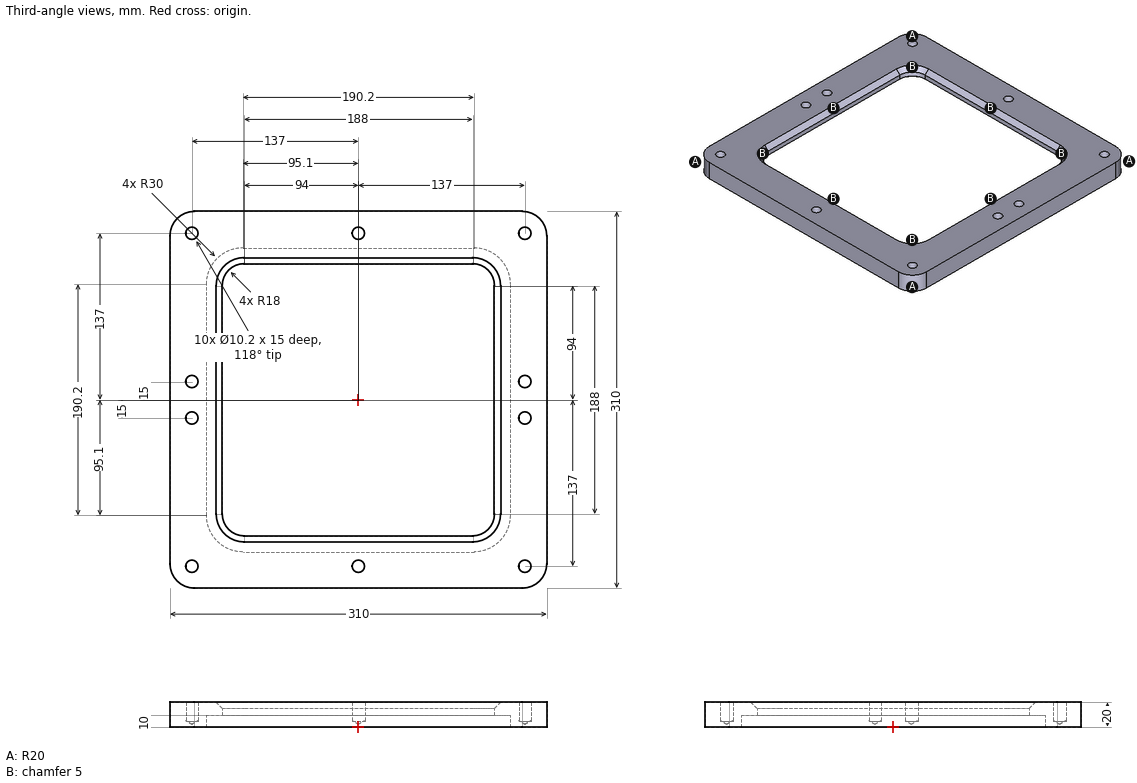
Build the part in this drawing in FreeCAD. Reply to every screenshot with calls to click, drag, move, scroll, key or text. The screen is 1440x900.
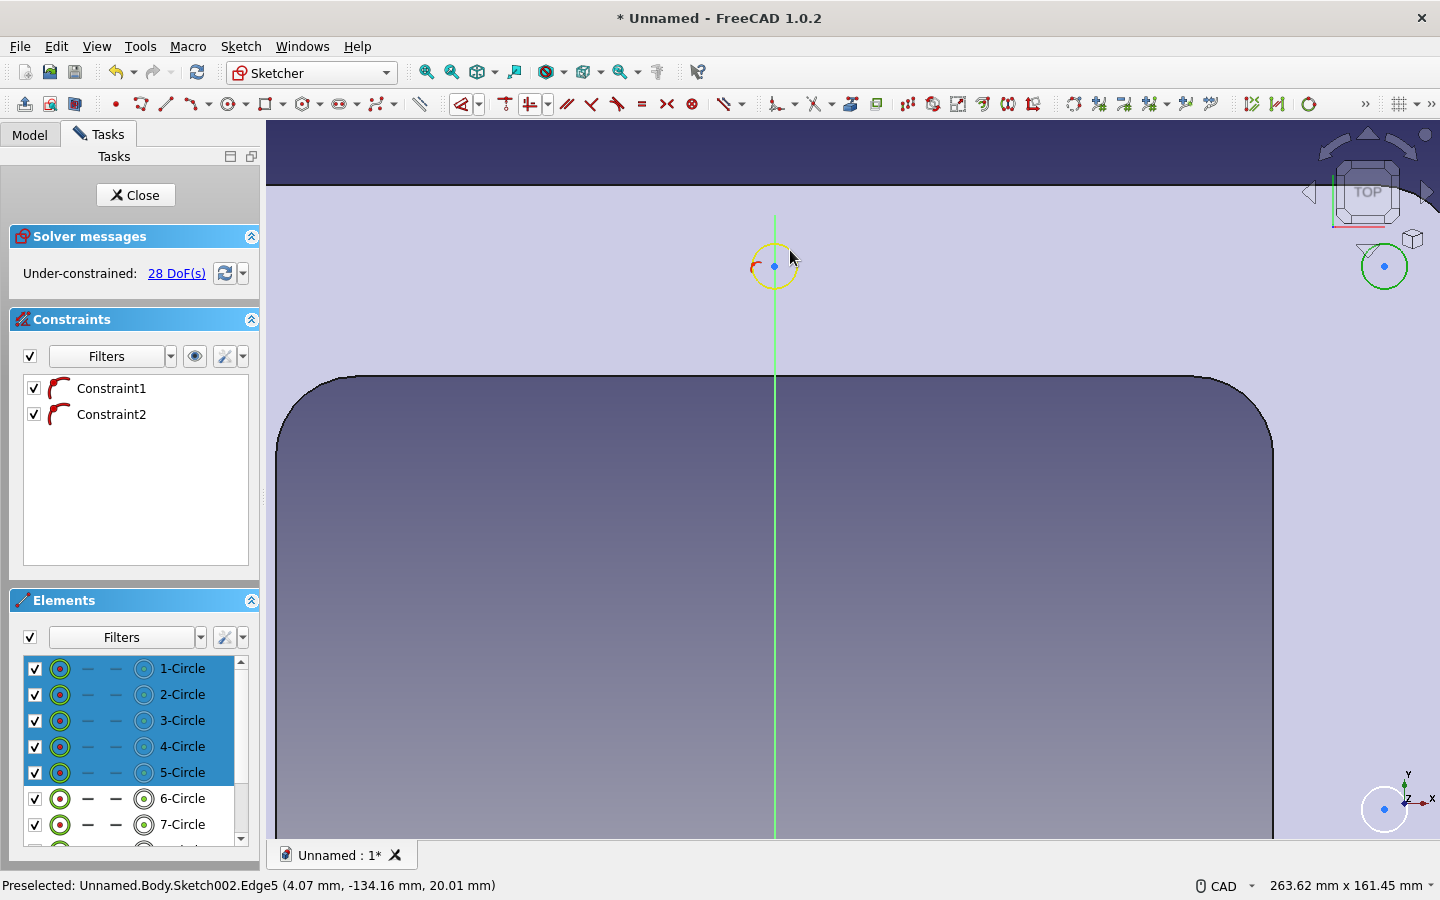
click(790, 250)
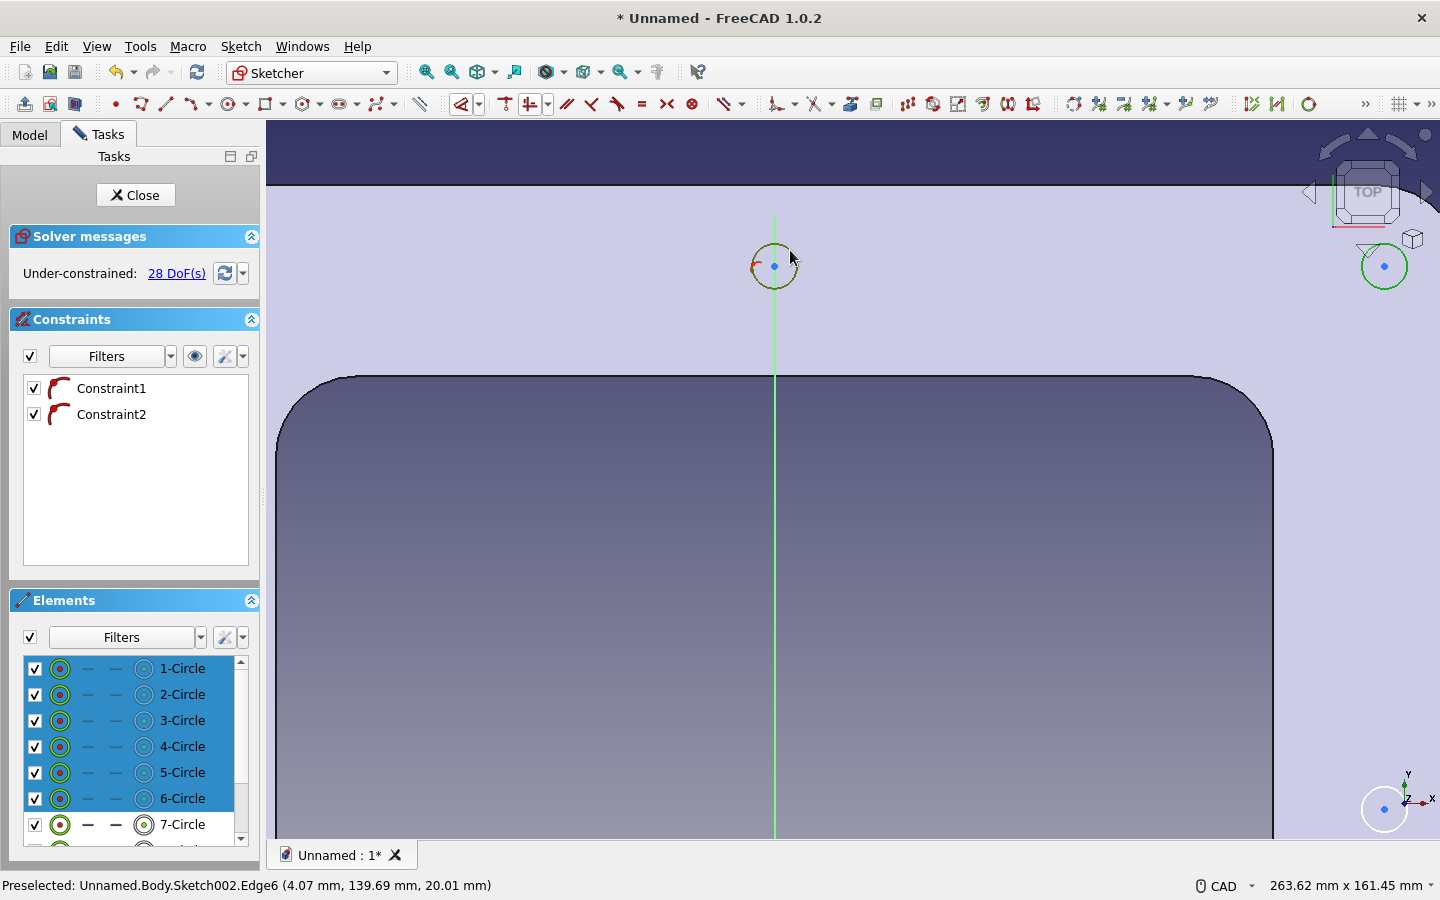
scroll(790, 249, down, 5)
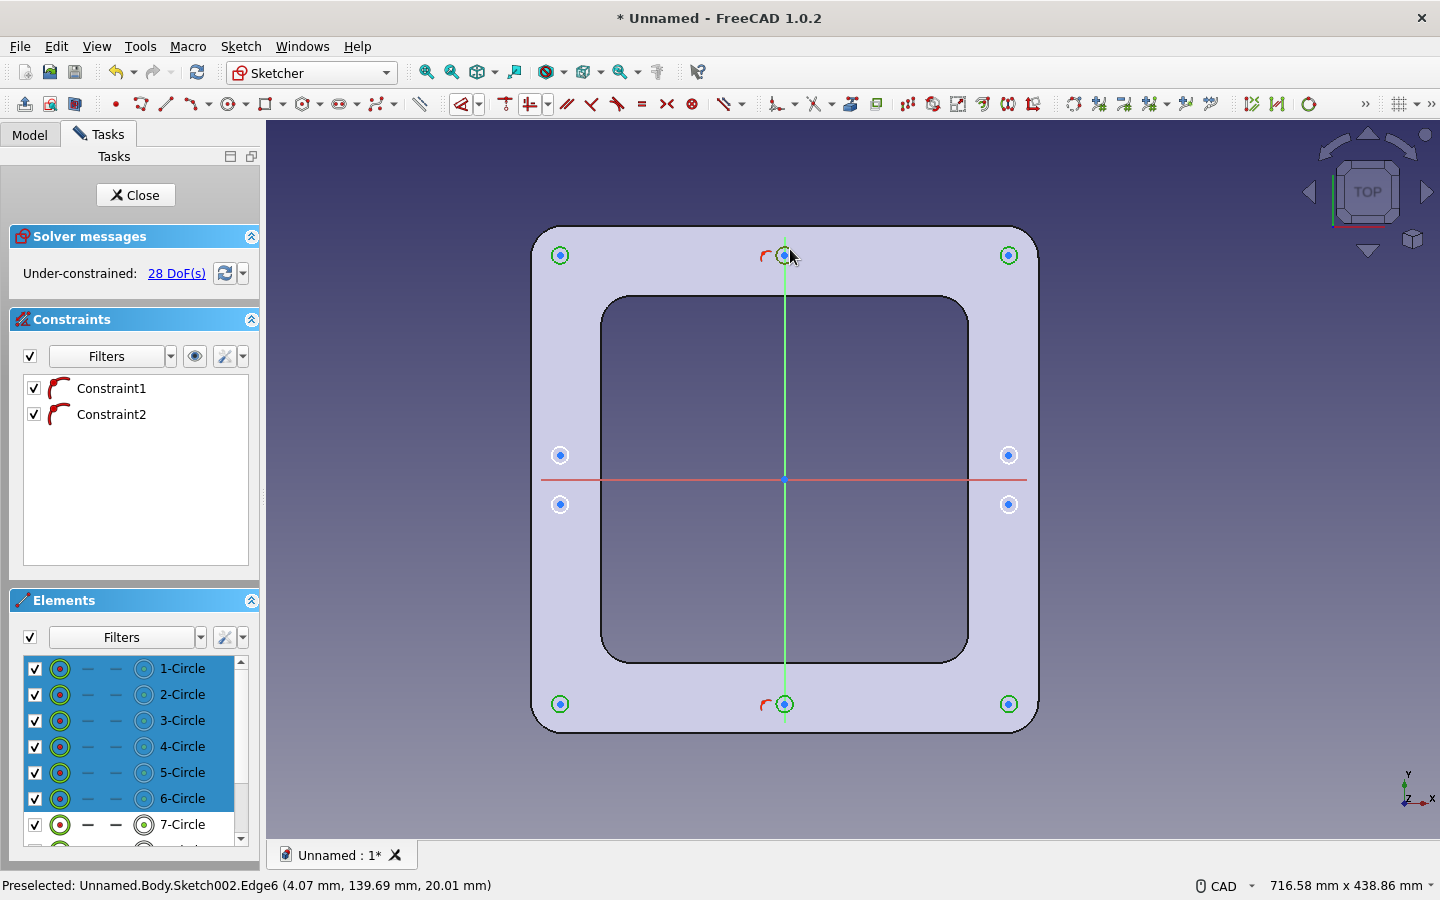
scroll(566, 449, up, 3)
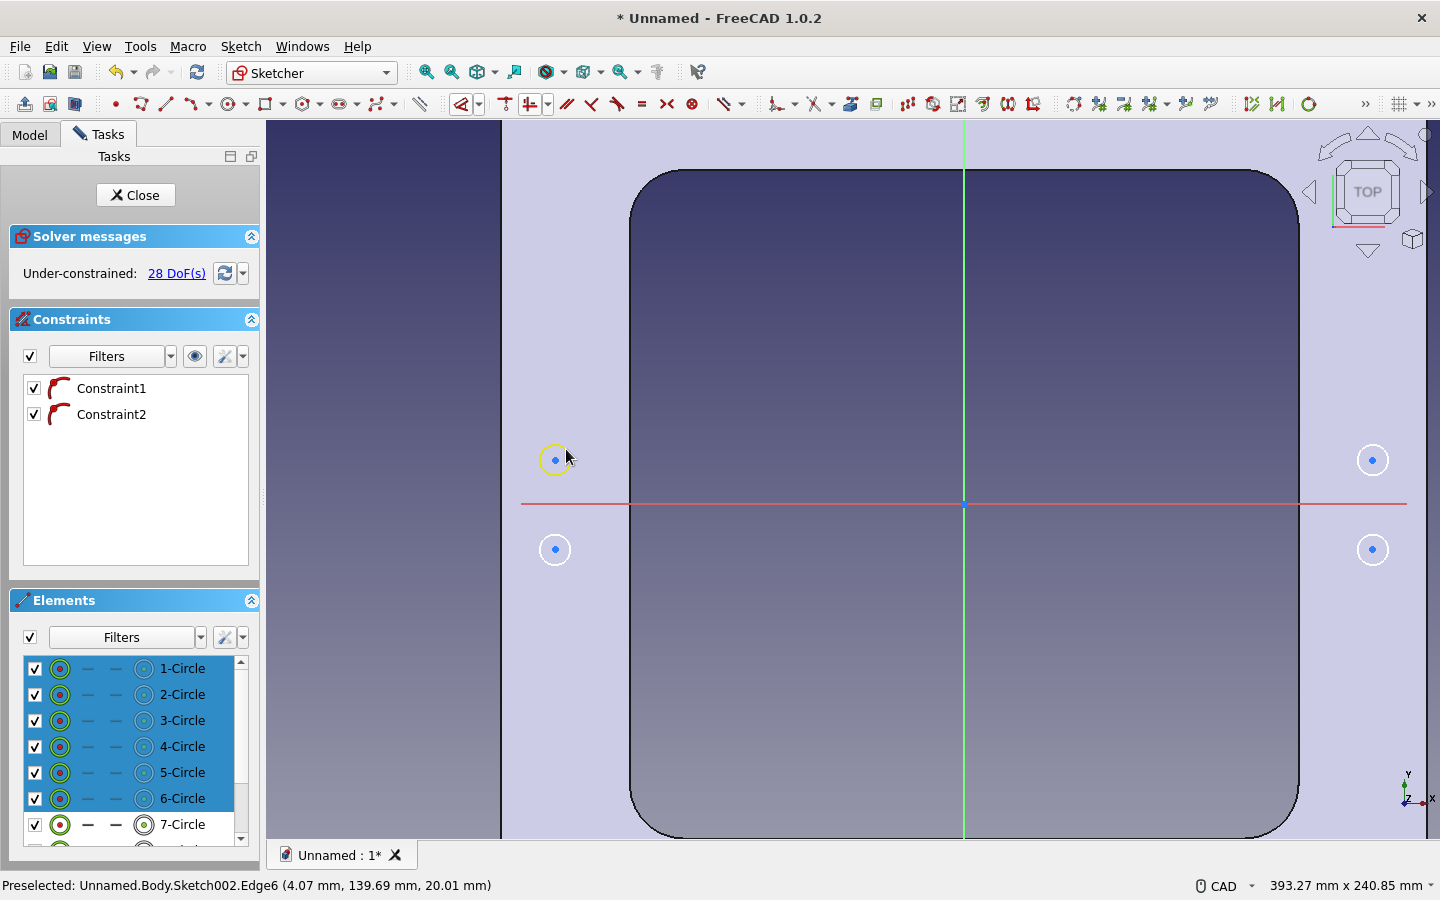
click(566, 449)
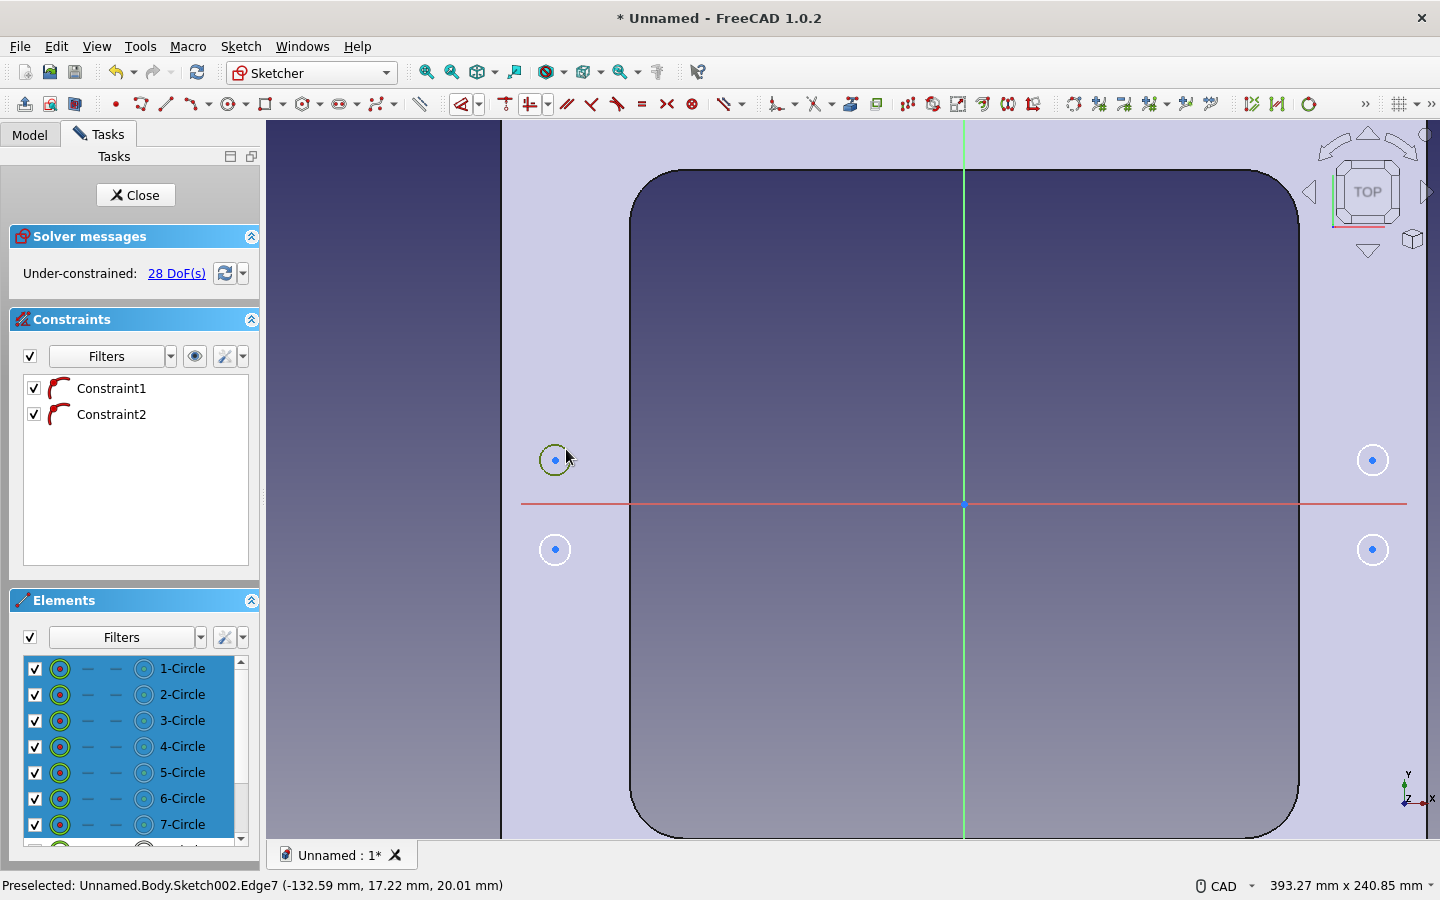
click(566, 539)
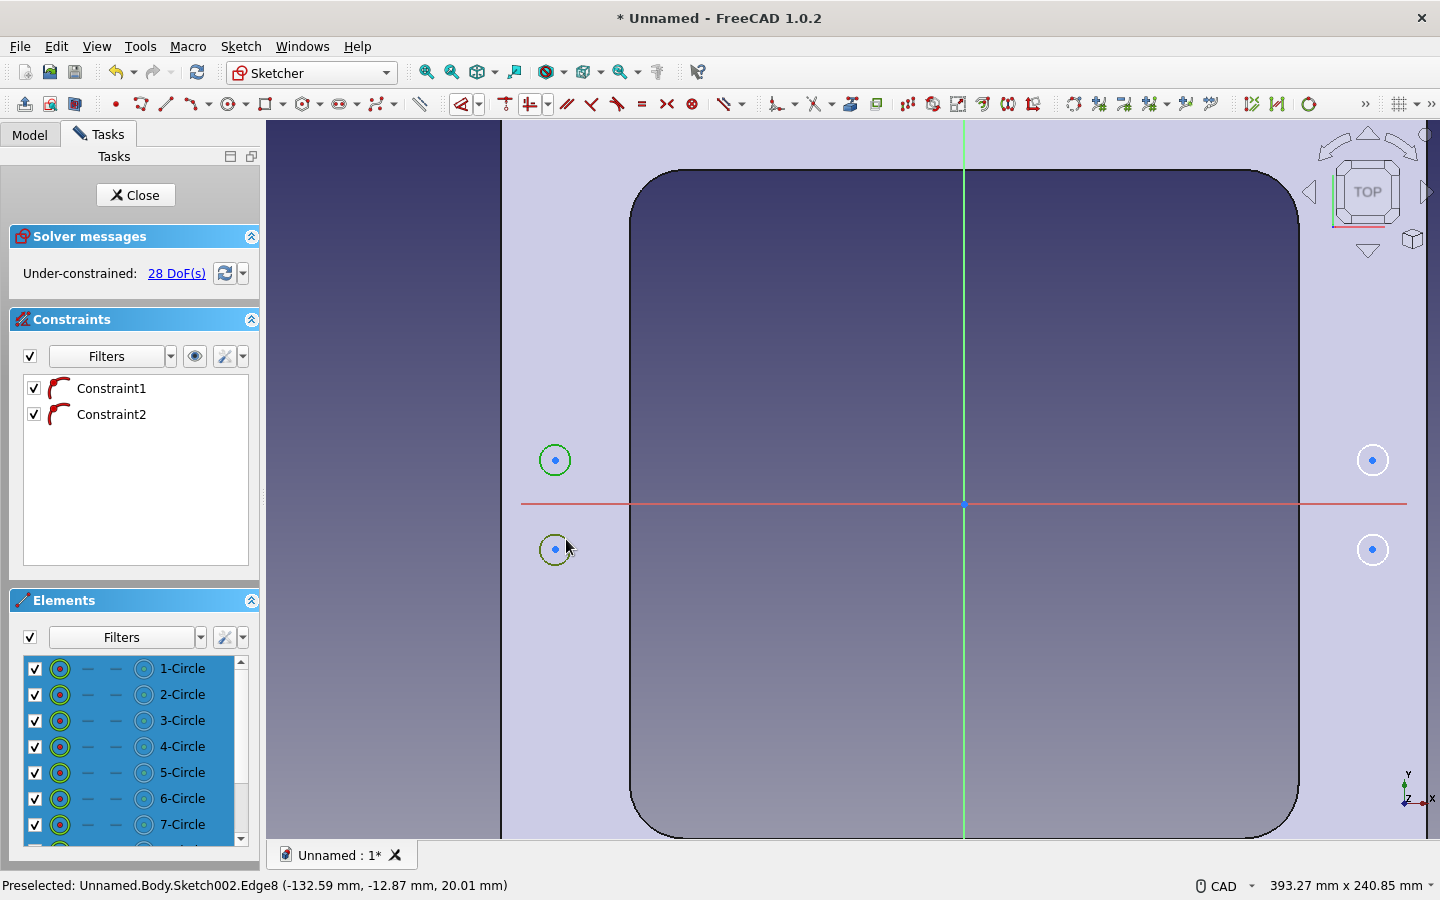
scroll(566, 449, down, 3)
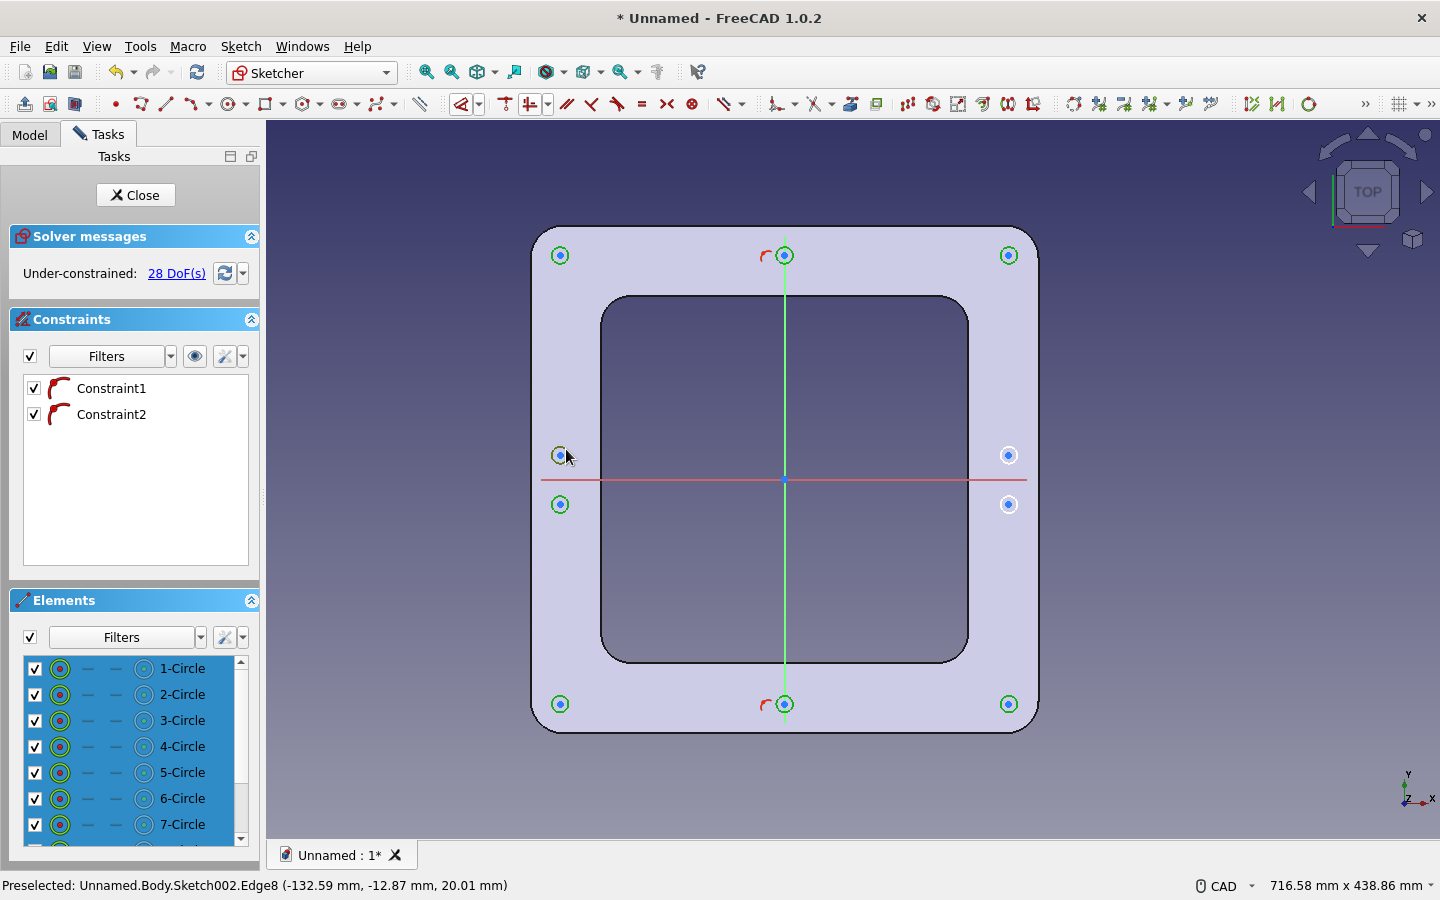
scroll(1015, 449, up, 3)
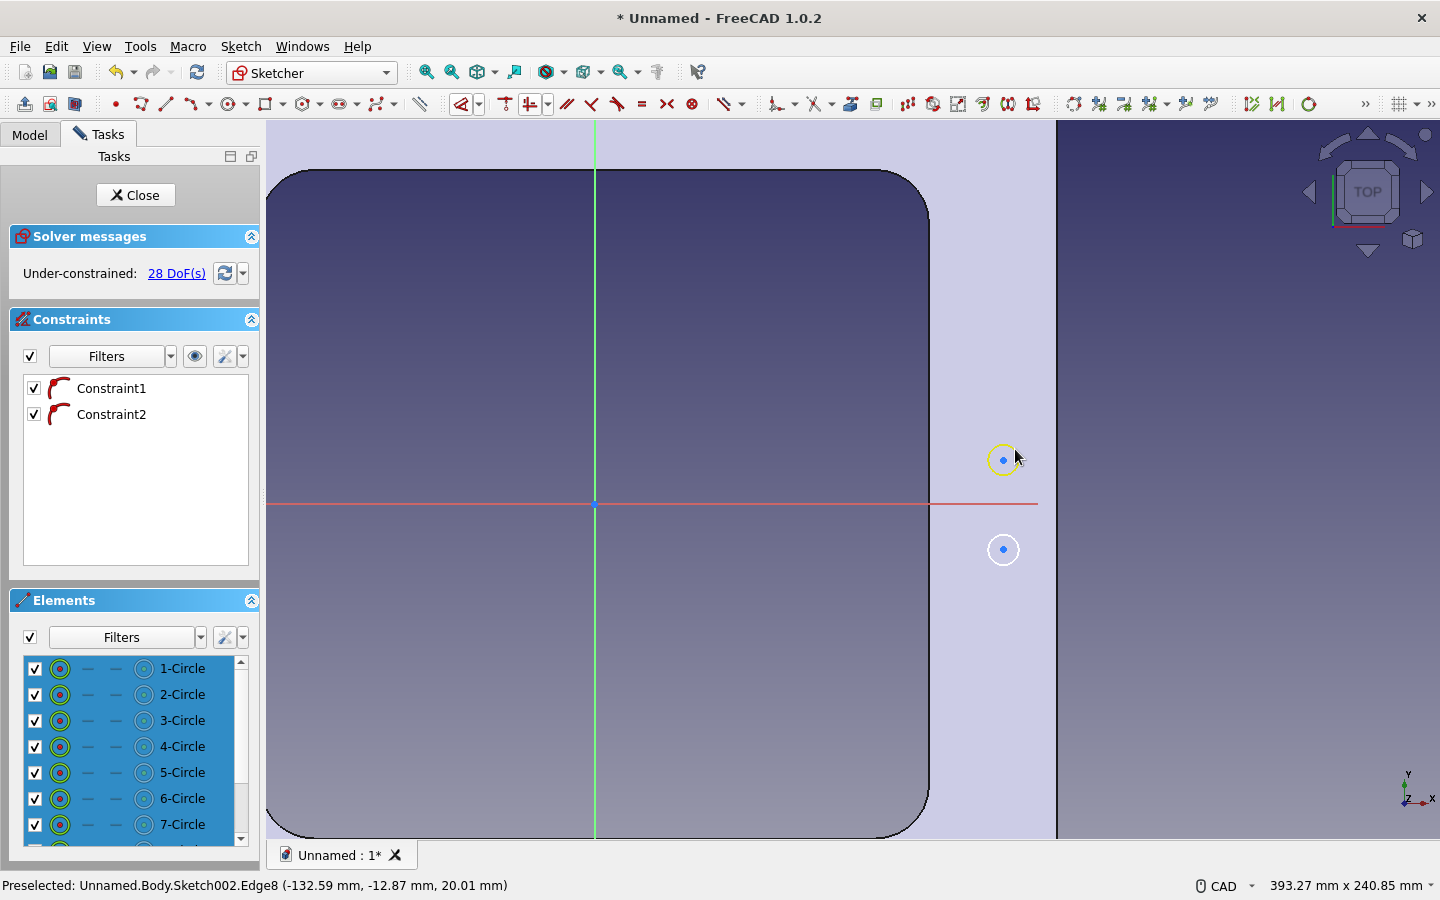
click(1014, 449)